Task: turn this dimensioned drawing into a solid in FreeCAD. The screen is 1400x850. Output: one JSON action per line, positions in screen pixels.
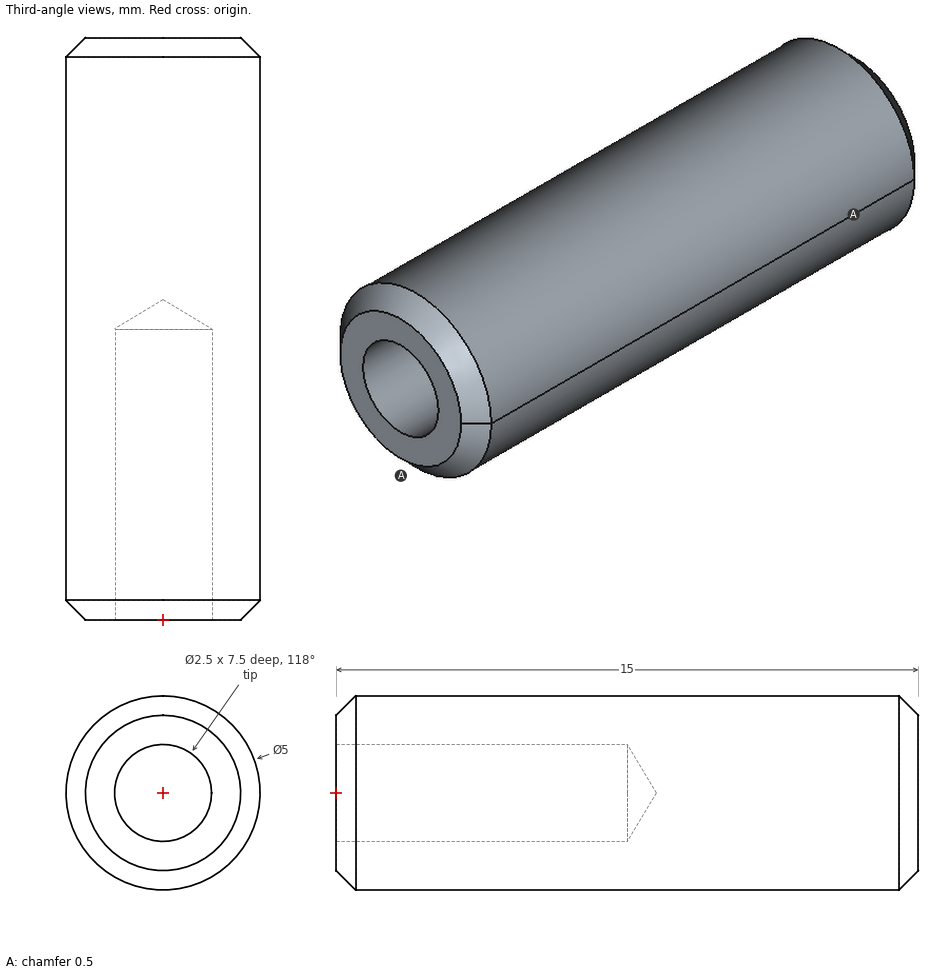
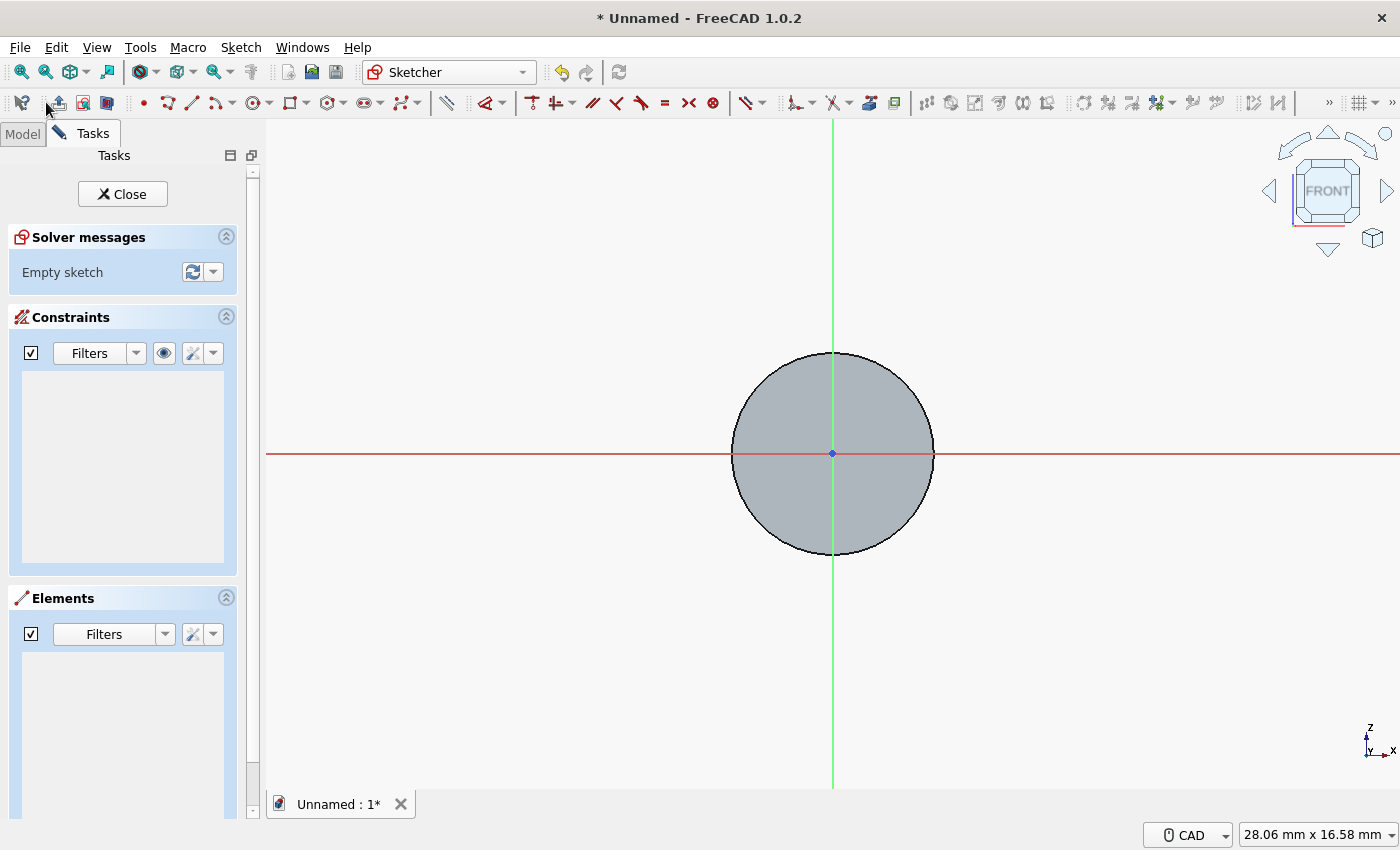
{"action": "scroll", "coordinate": [855, 454], "scroll_direction": "up", "scroll_amount": 7}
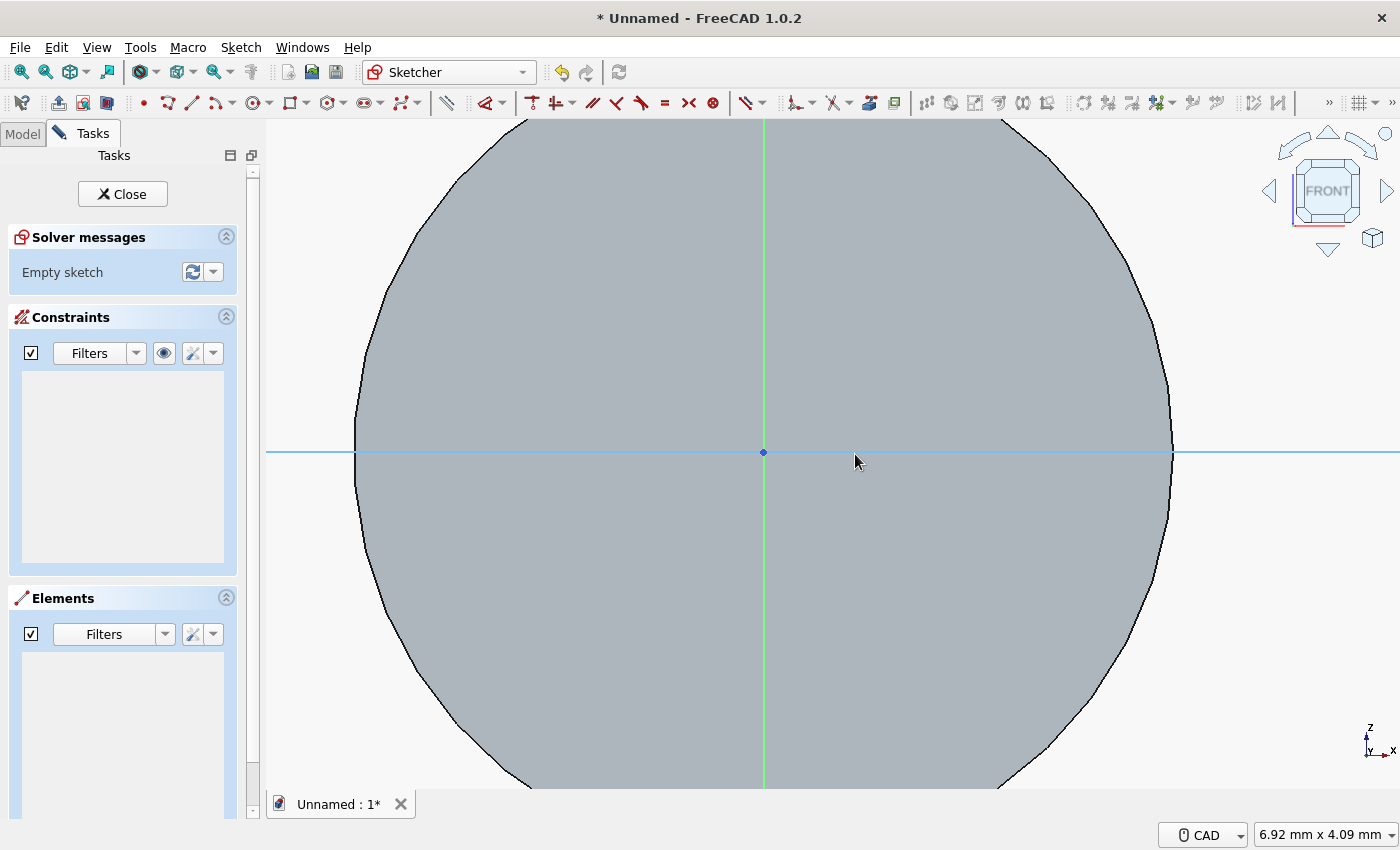
{"action": "left_click", "coordinate": [254, 104]}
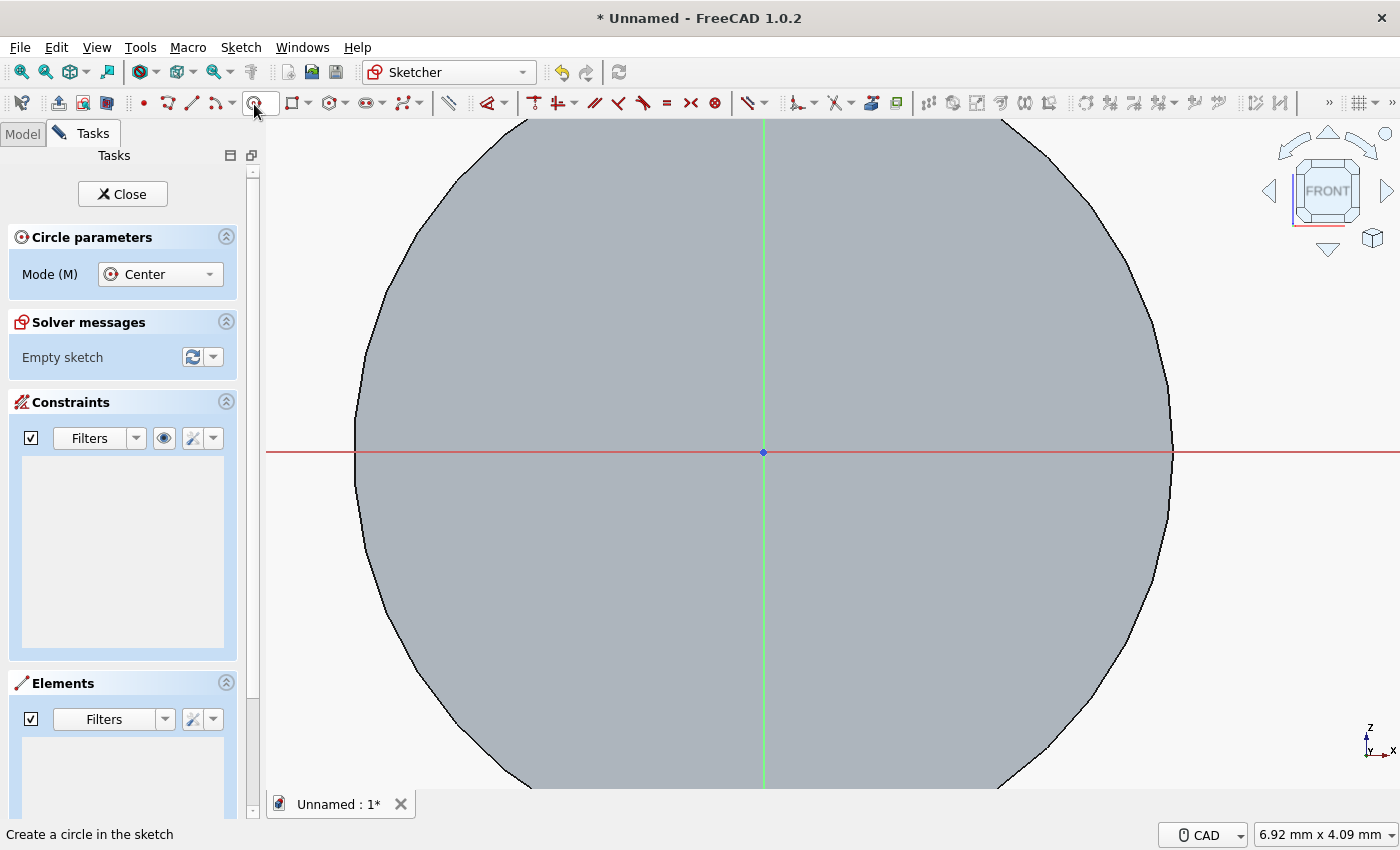
{"action": "left_click", "coordinate": [764, 452]}
{"action": "mouse_move", "coordinate": [908, 308]}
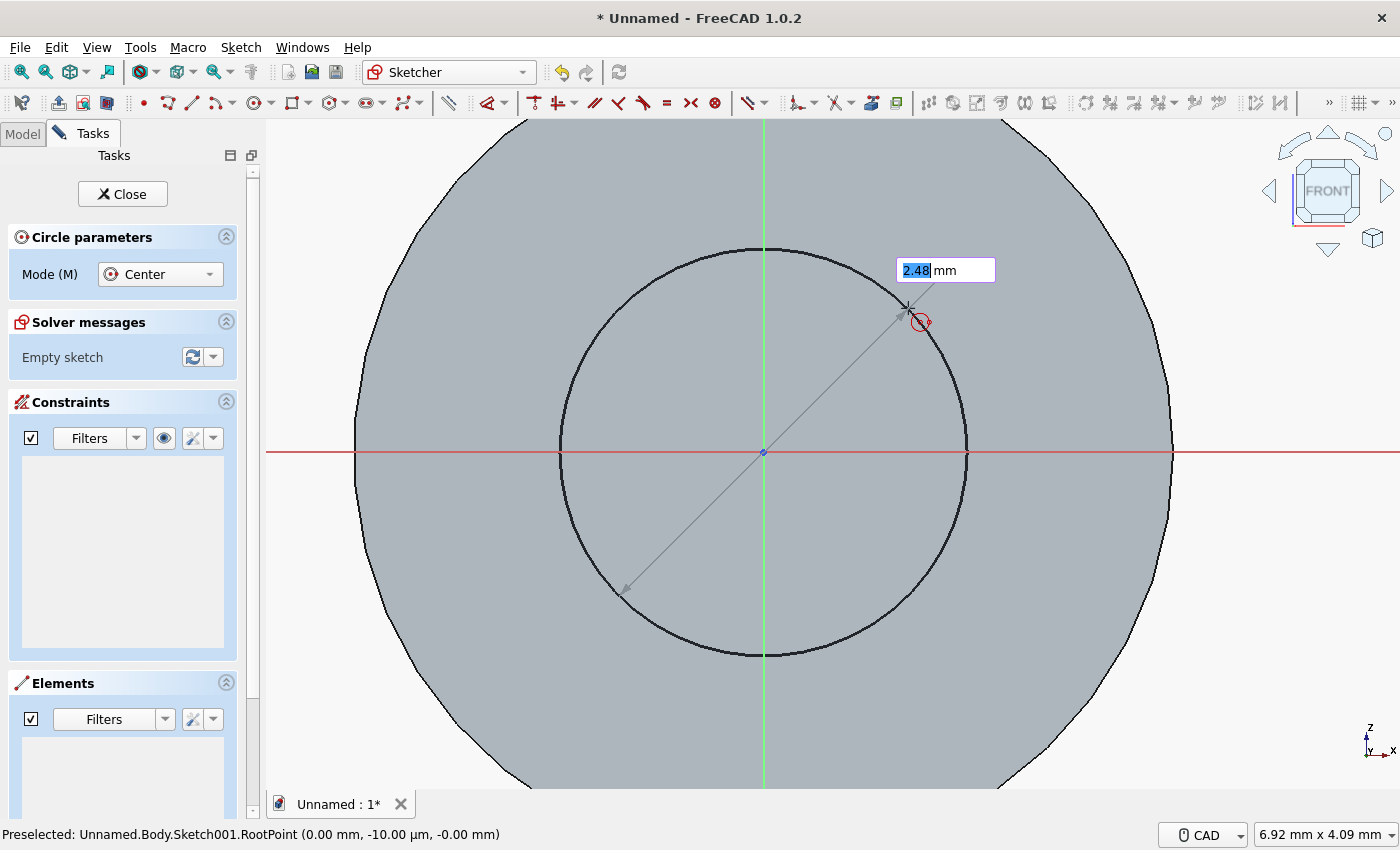
{"action": "type", "text": "2.5"}
{"action": "key", "text": "Return"}
{"action": "key", "text": "Escape"}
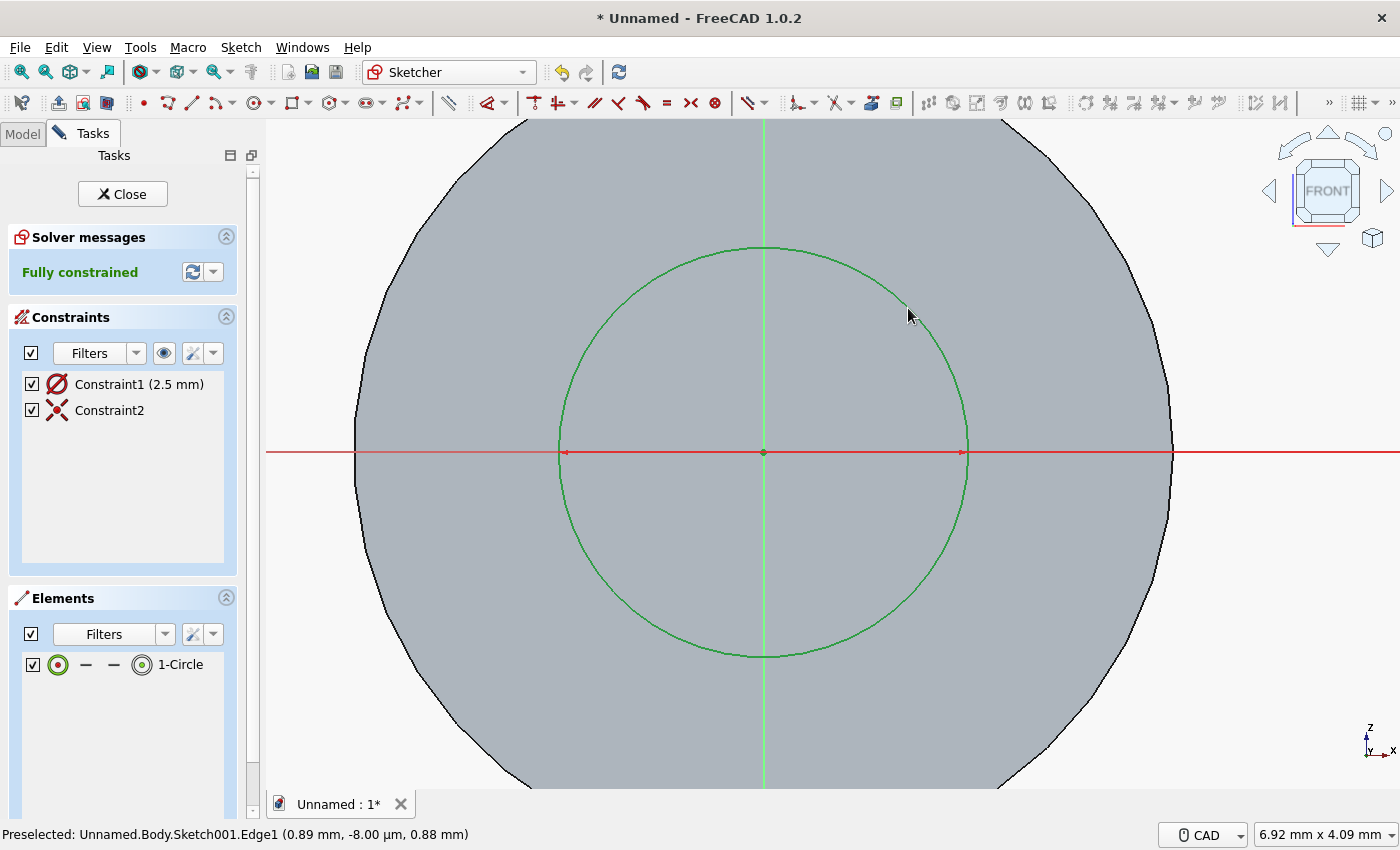
{"action": "left_click", "coordinate": [123, 194]}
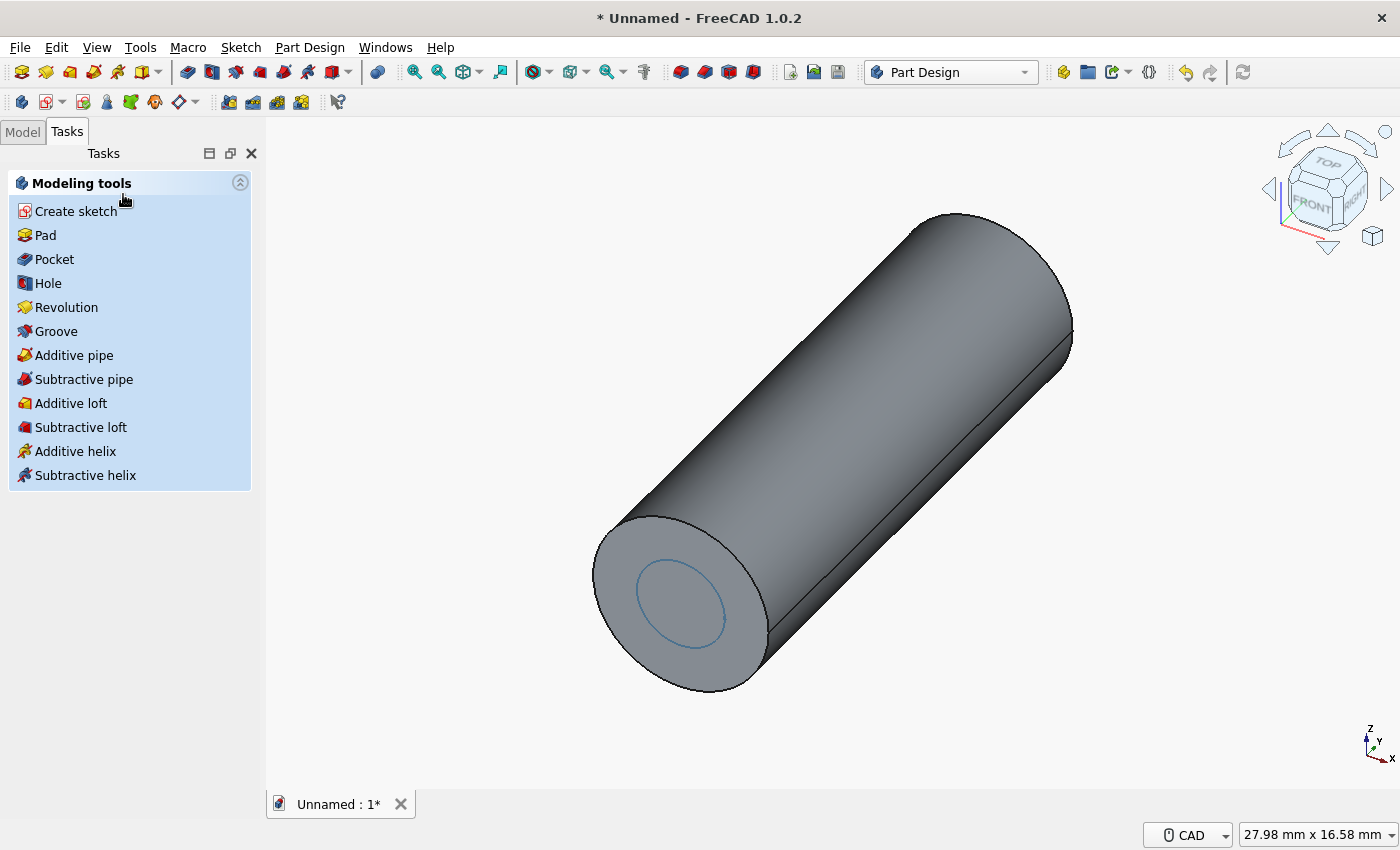
{"action": "left_click", "coordinate": [212, 72]}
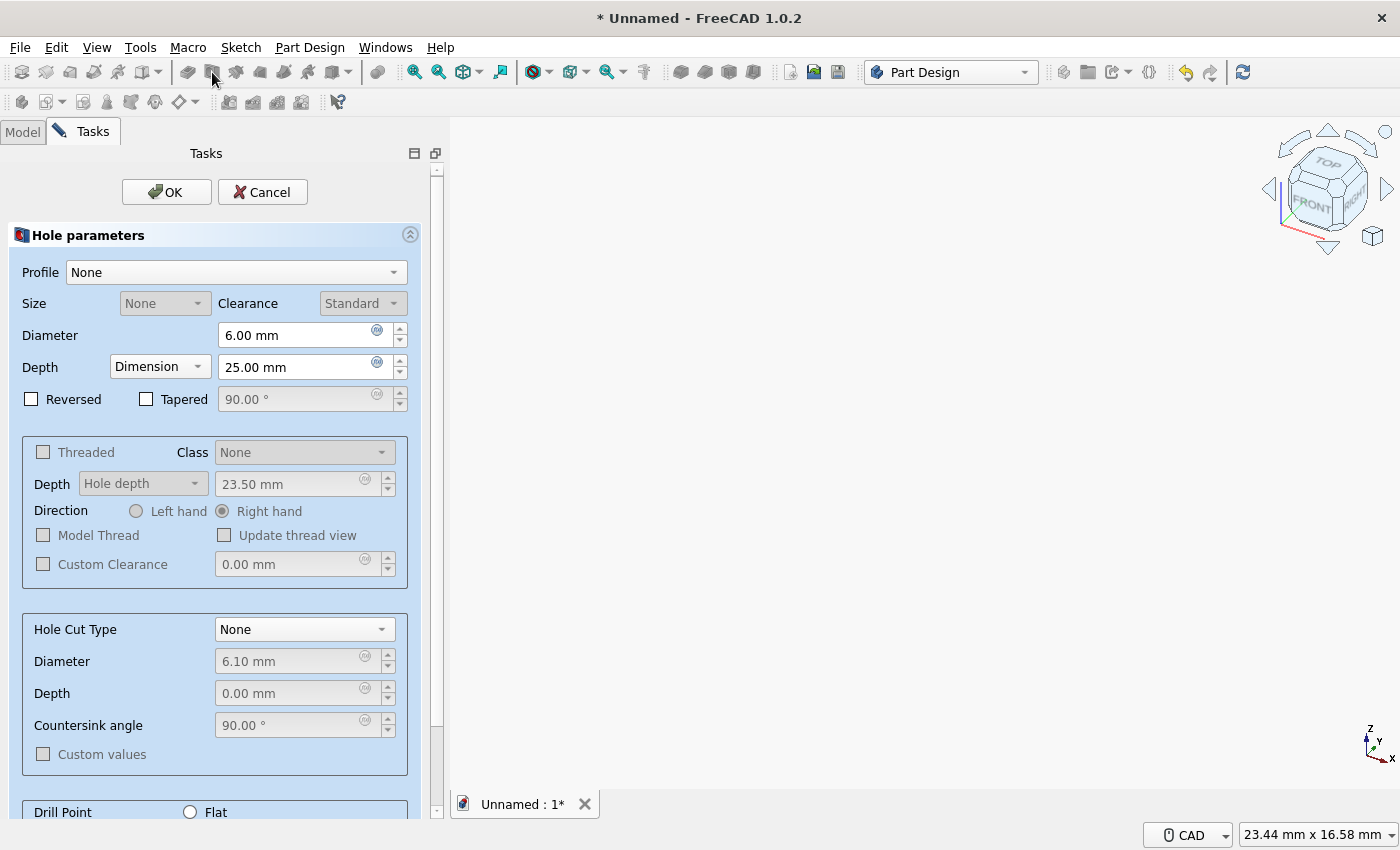
{"action": "triple_click", "coordinate": [305, 335]}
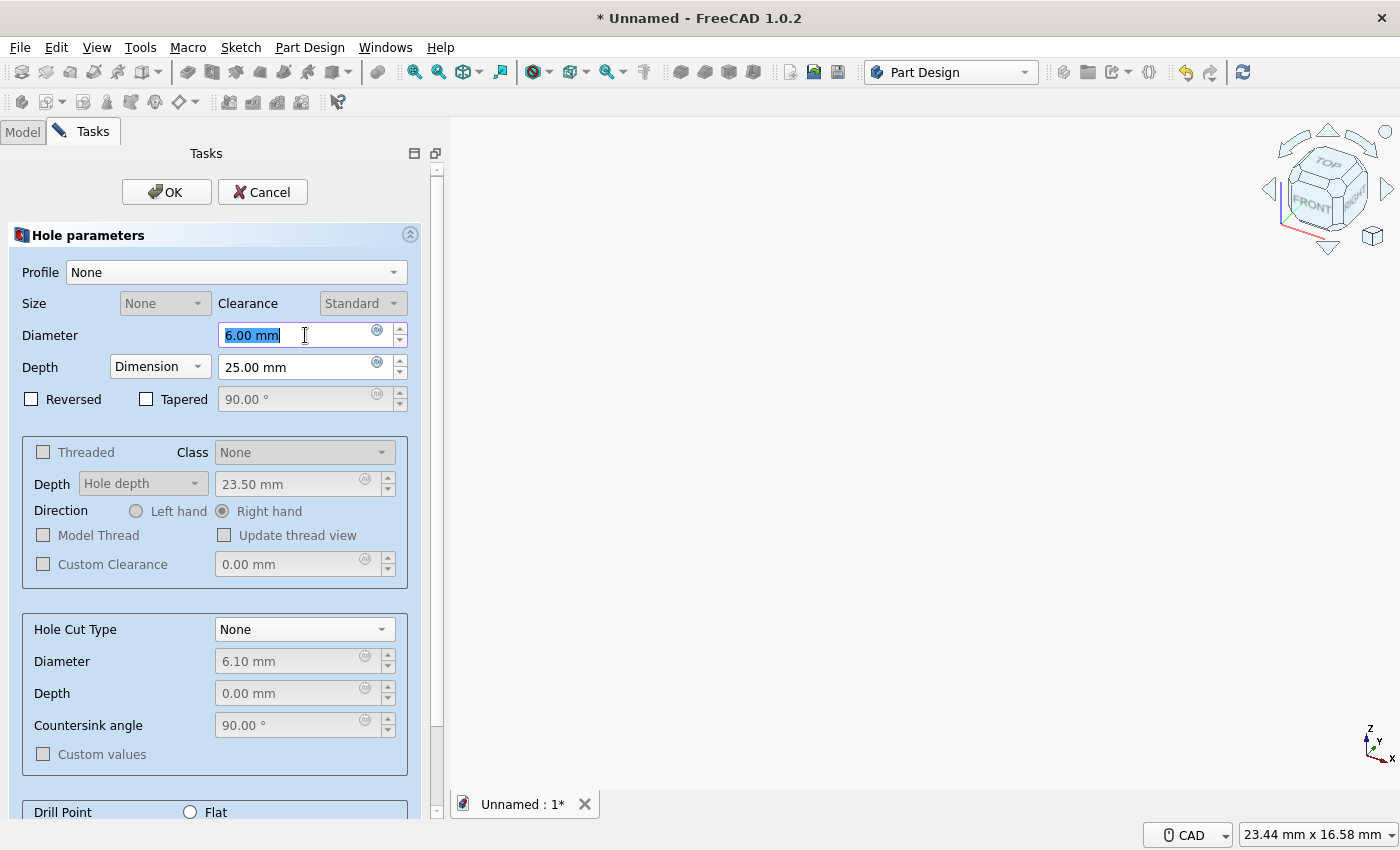
{"action": "type", "text": "2.5"}
{"action": "key", "text": "Tab"}